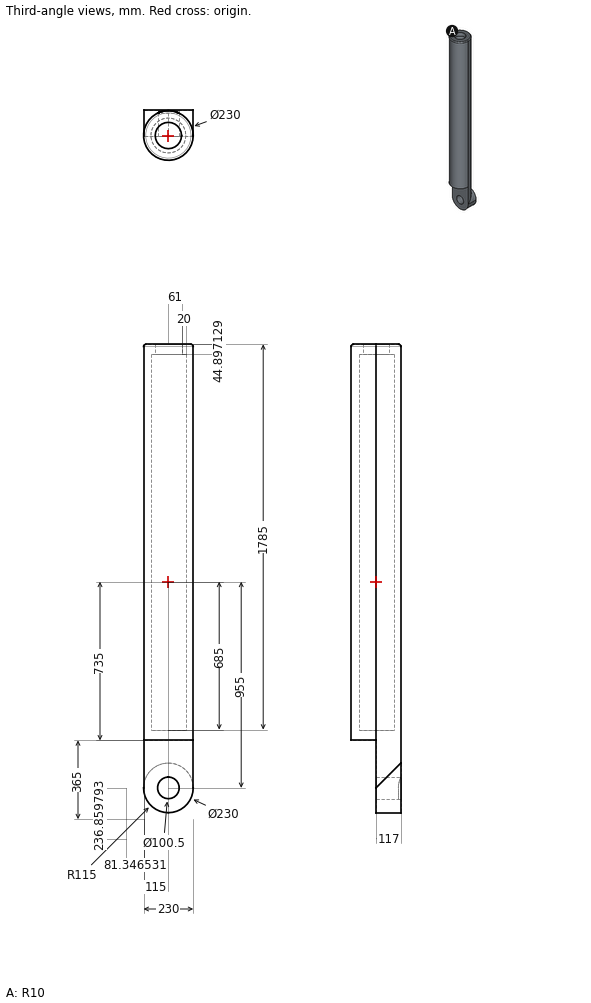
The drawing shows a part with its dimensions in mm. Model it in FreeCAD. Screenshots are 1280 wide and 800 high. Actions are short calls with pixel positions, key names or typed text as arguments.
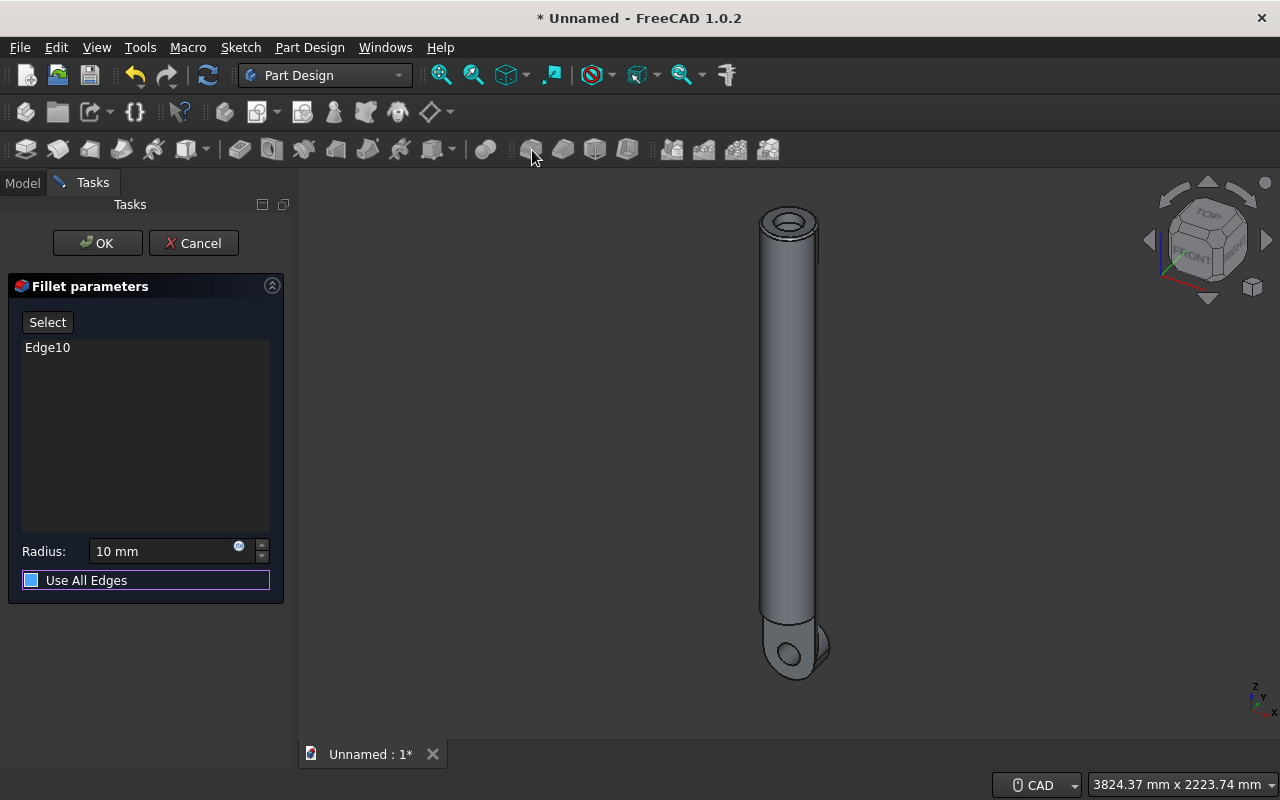
click(98, 243)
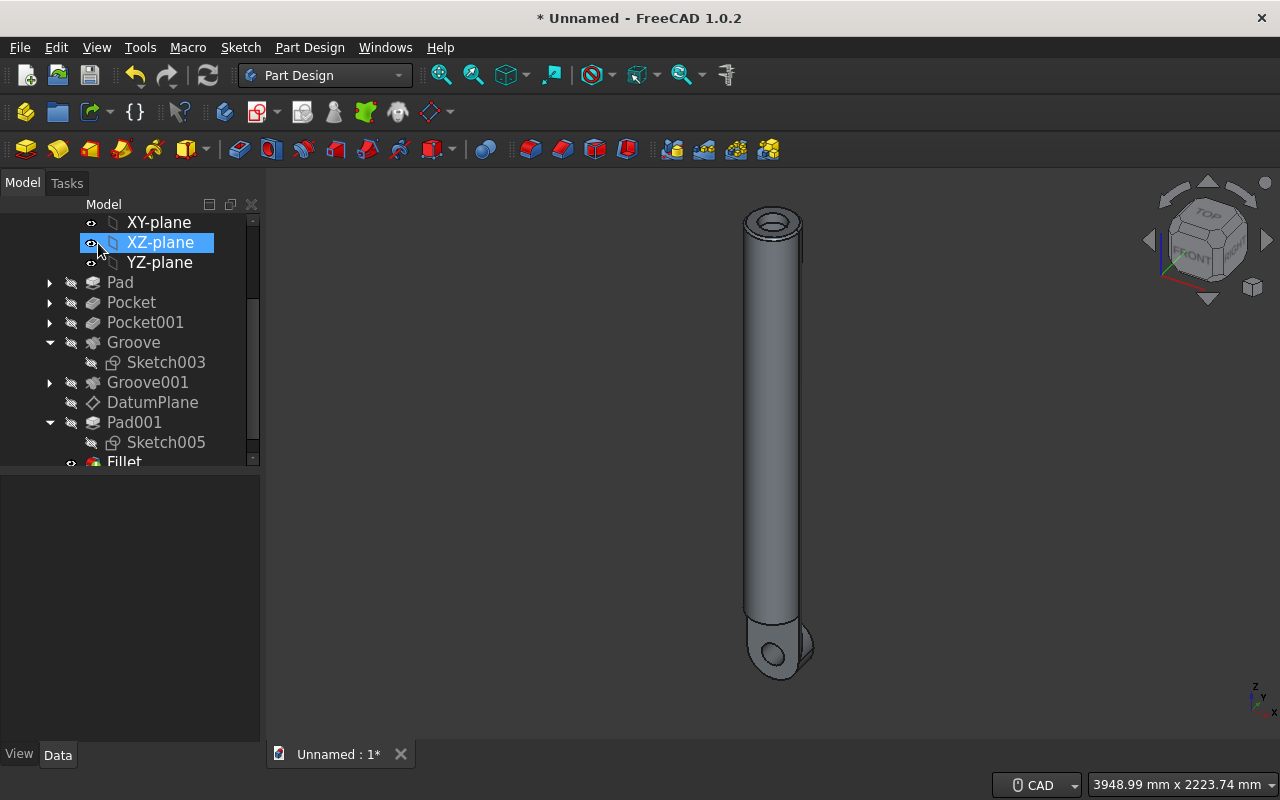
key(0)